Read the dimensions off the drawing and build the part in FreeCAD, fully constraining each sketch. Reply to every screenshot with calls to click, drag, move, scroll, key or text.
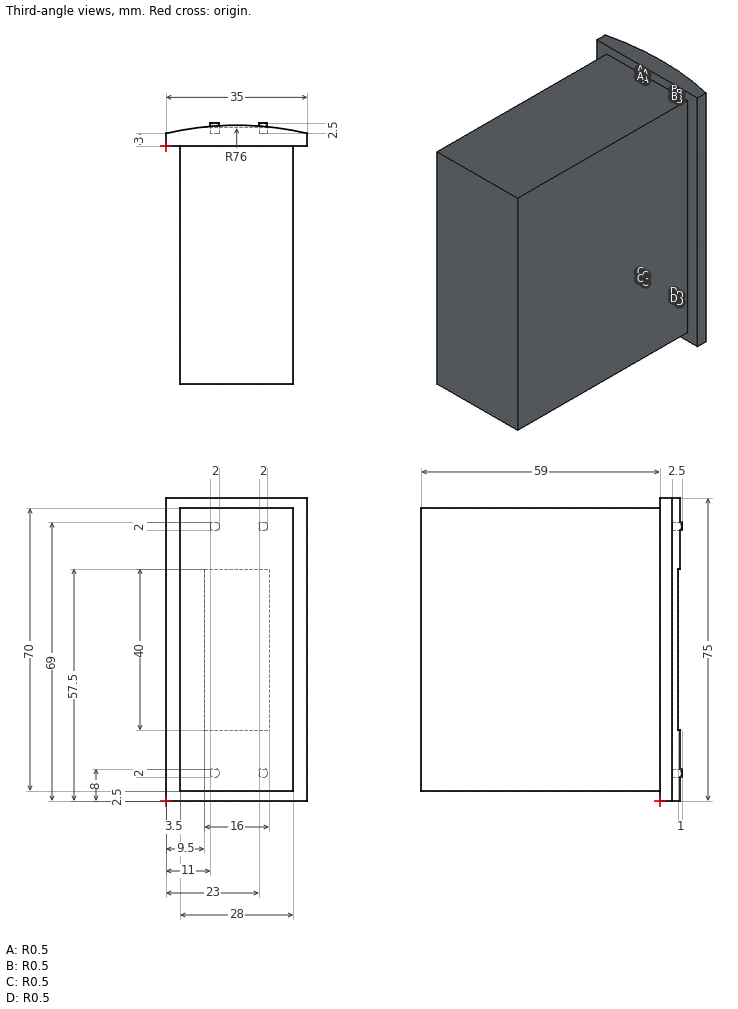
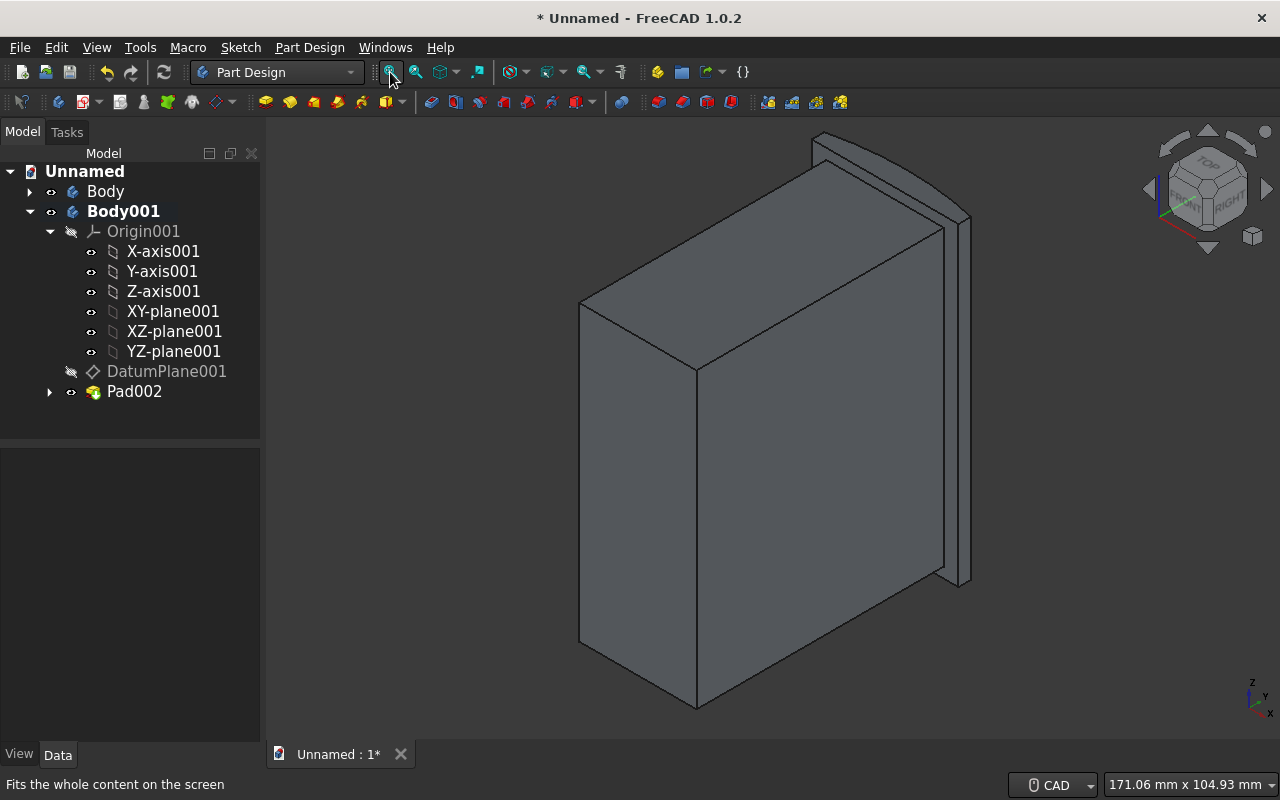
scroll(876, 184, up, 5)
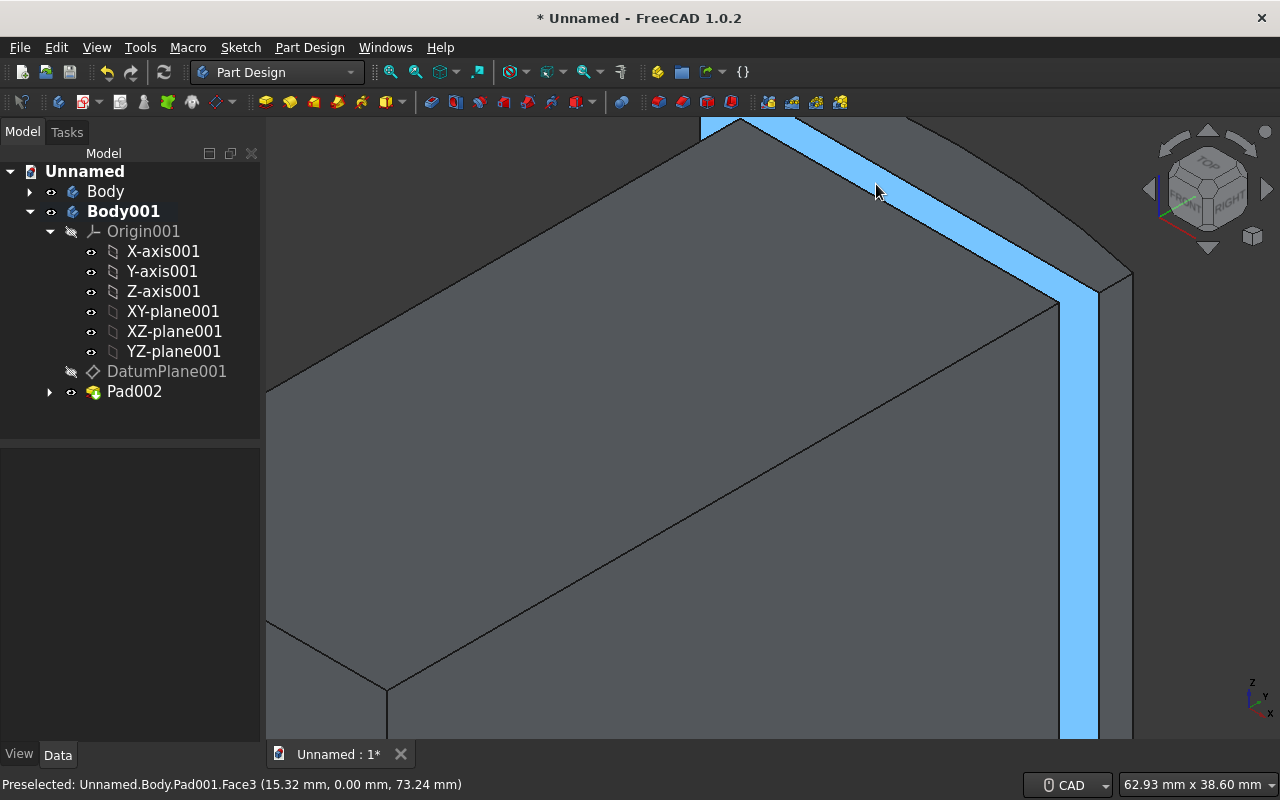
key(v)
key(f)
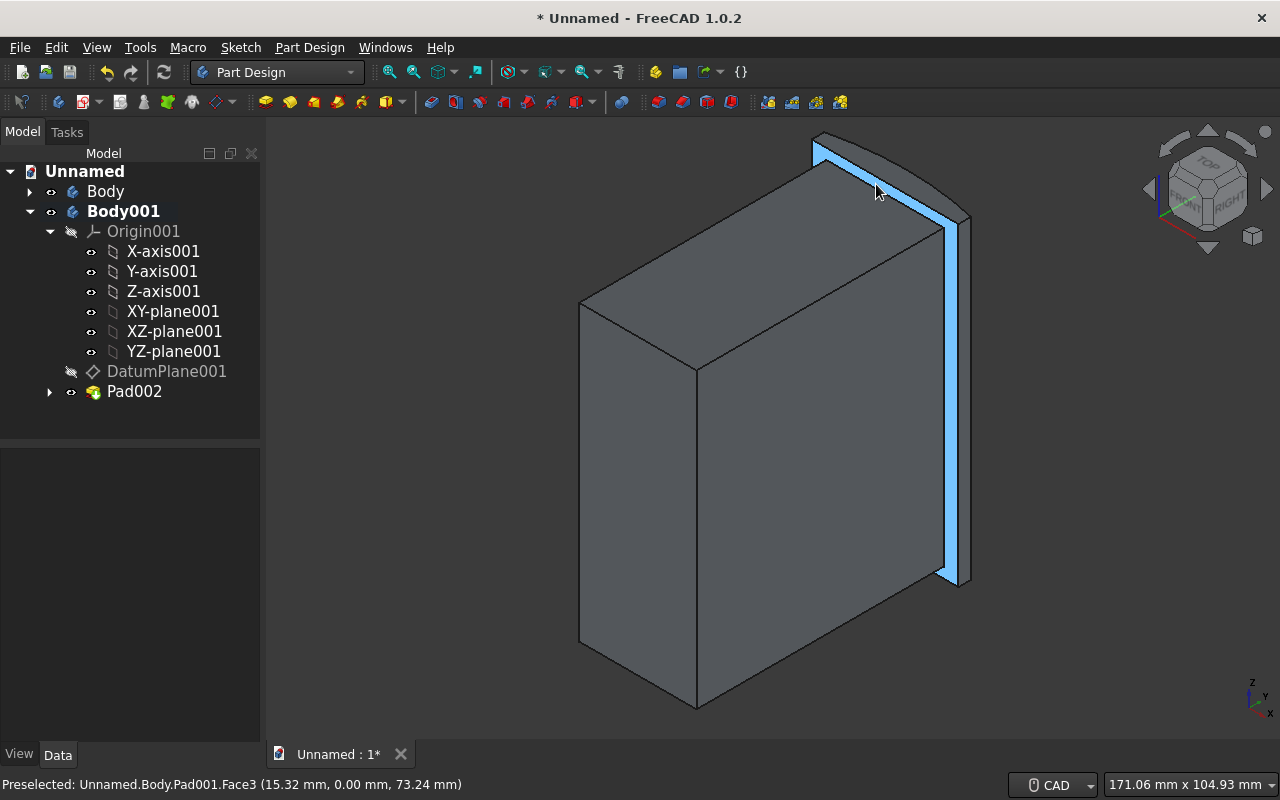
key(2)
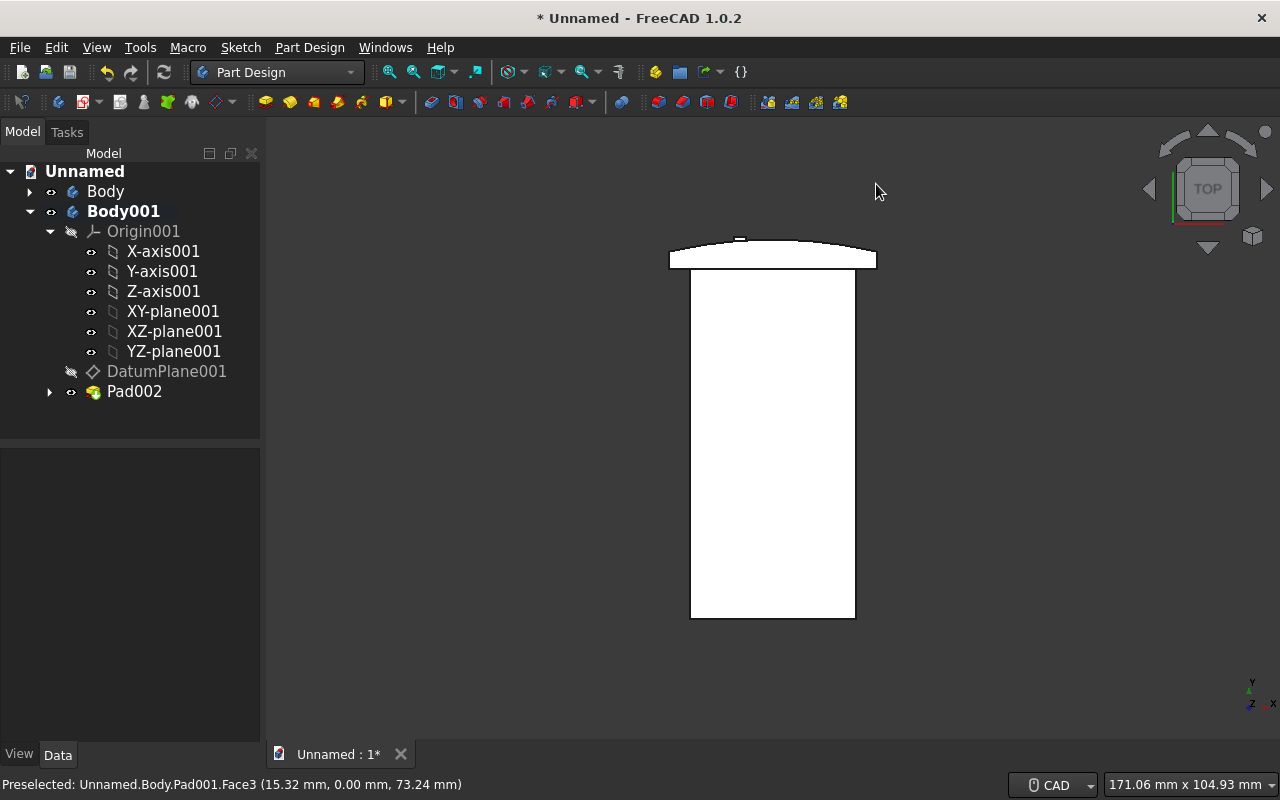
key(v)
key(f)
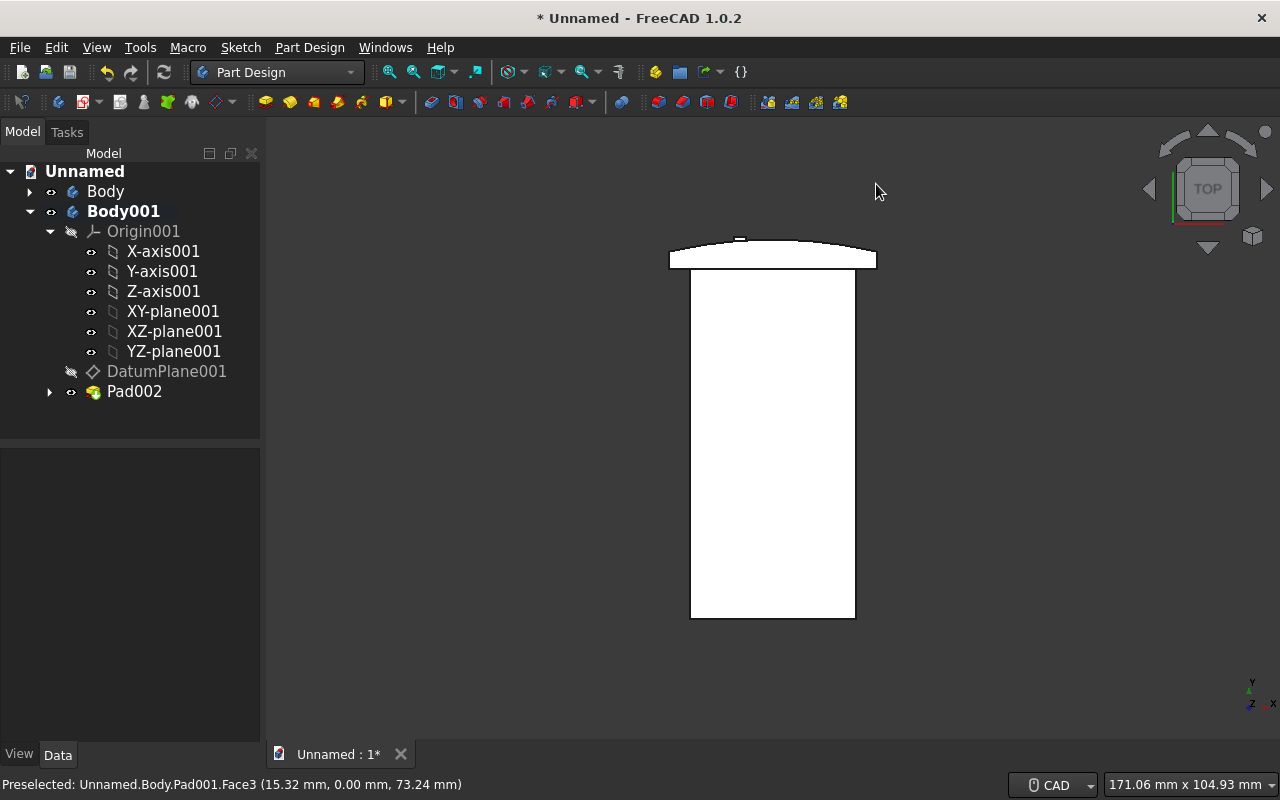
scroll(734, 243, up, 5)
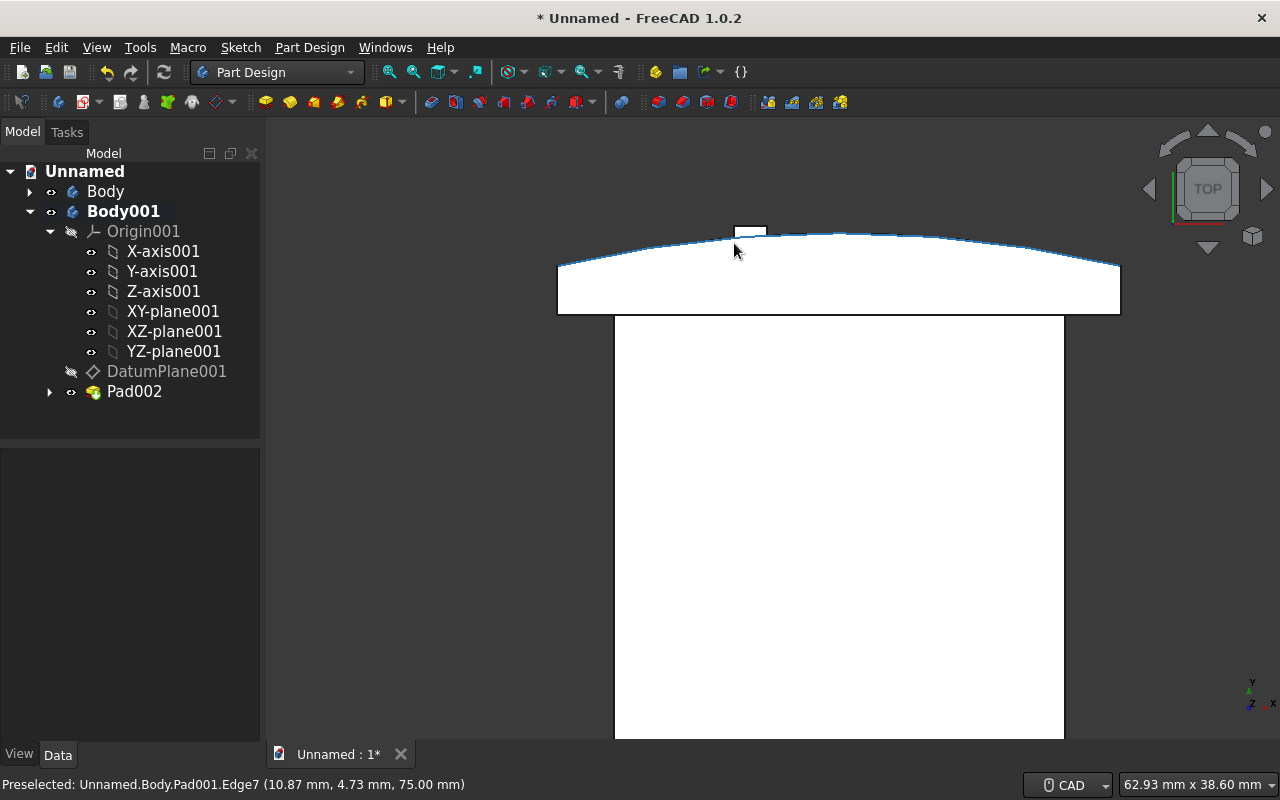
key(v)
key(f)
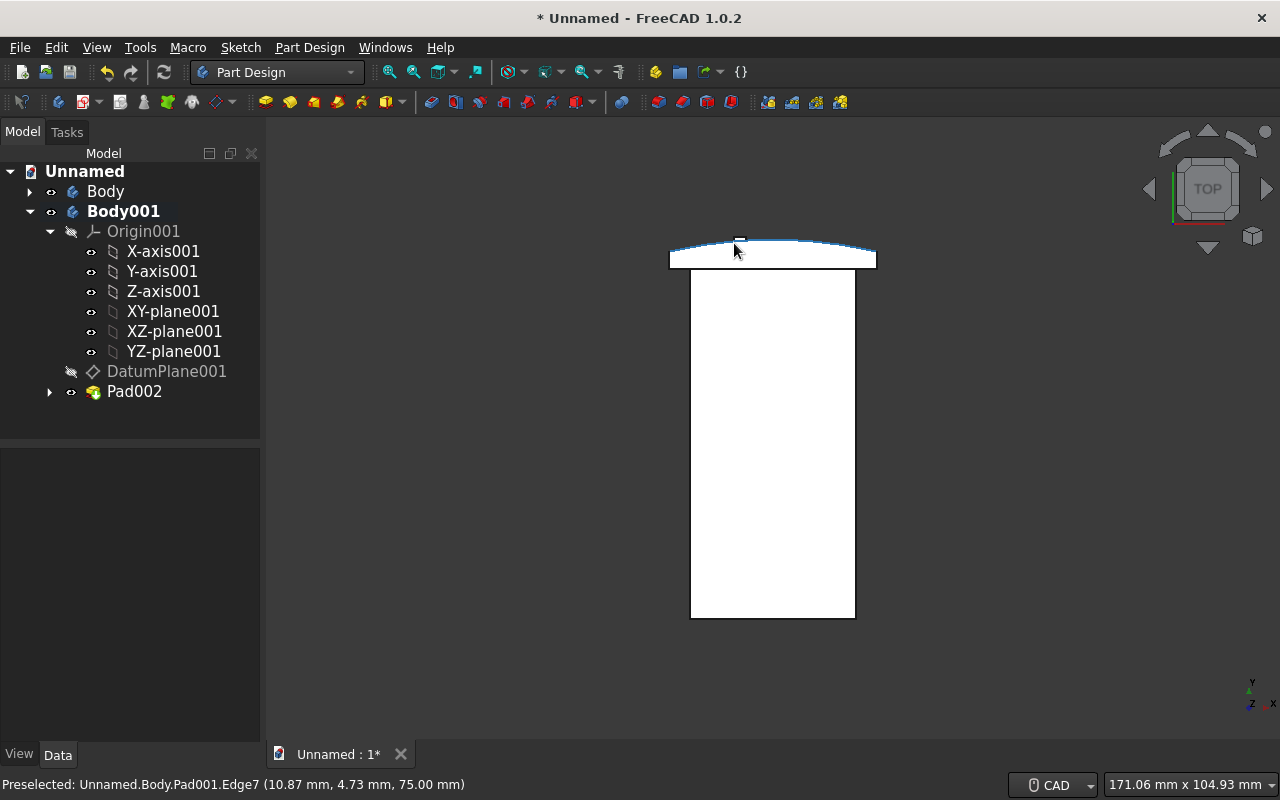
key(1)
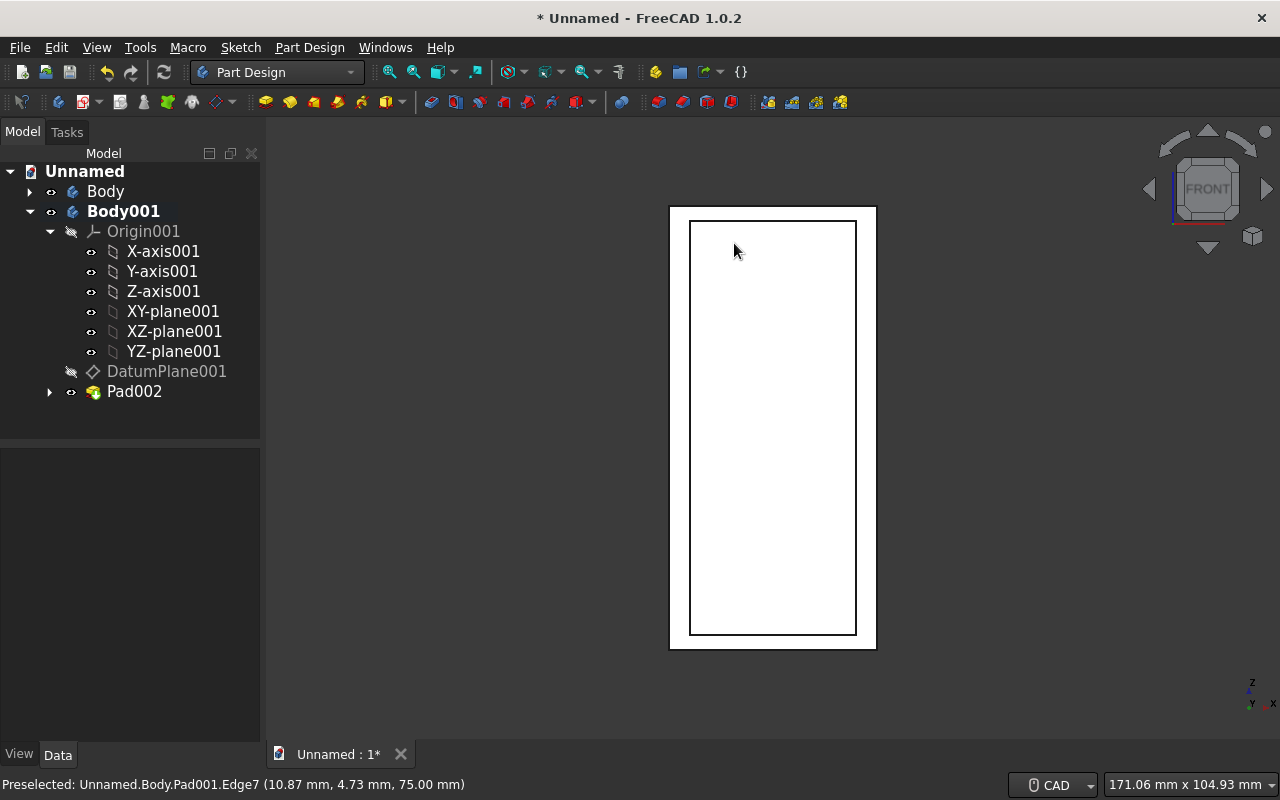
click(390, 72)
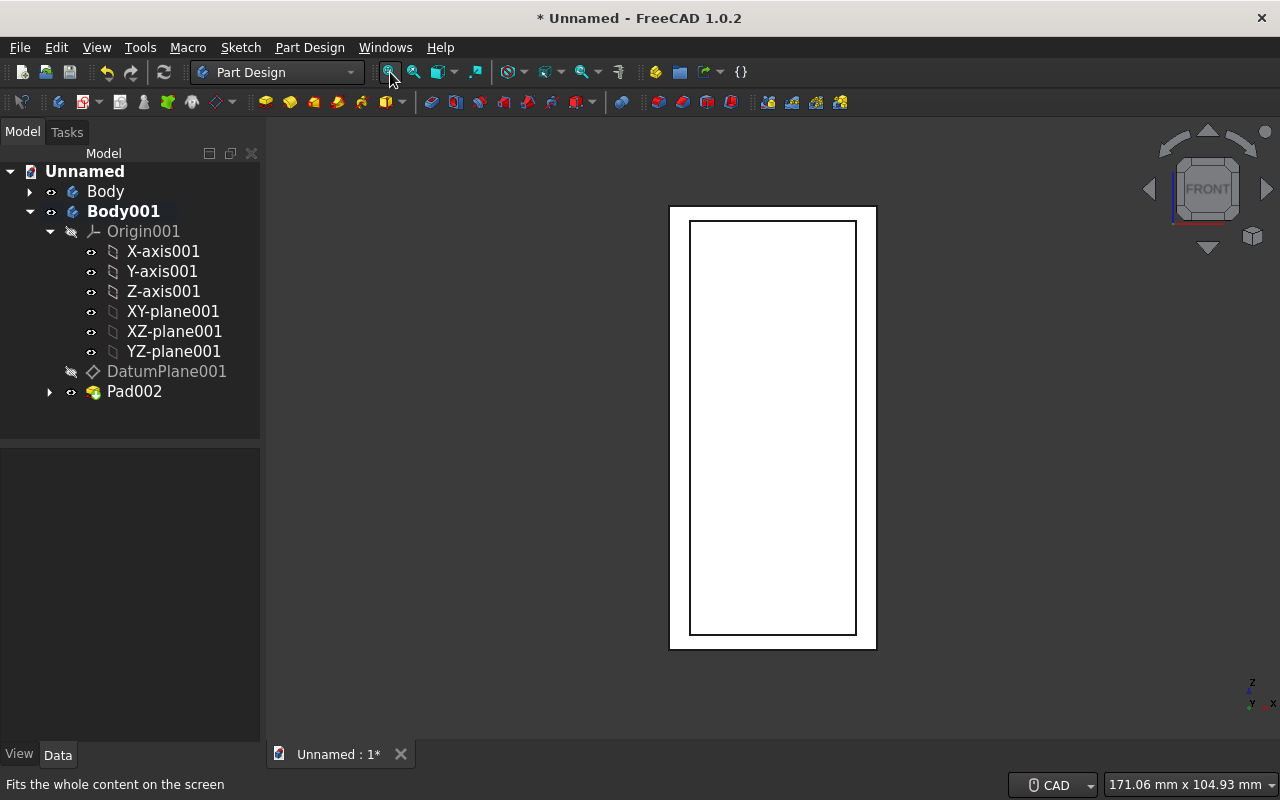
scroll(734, 240, up, 5)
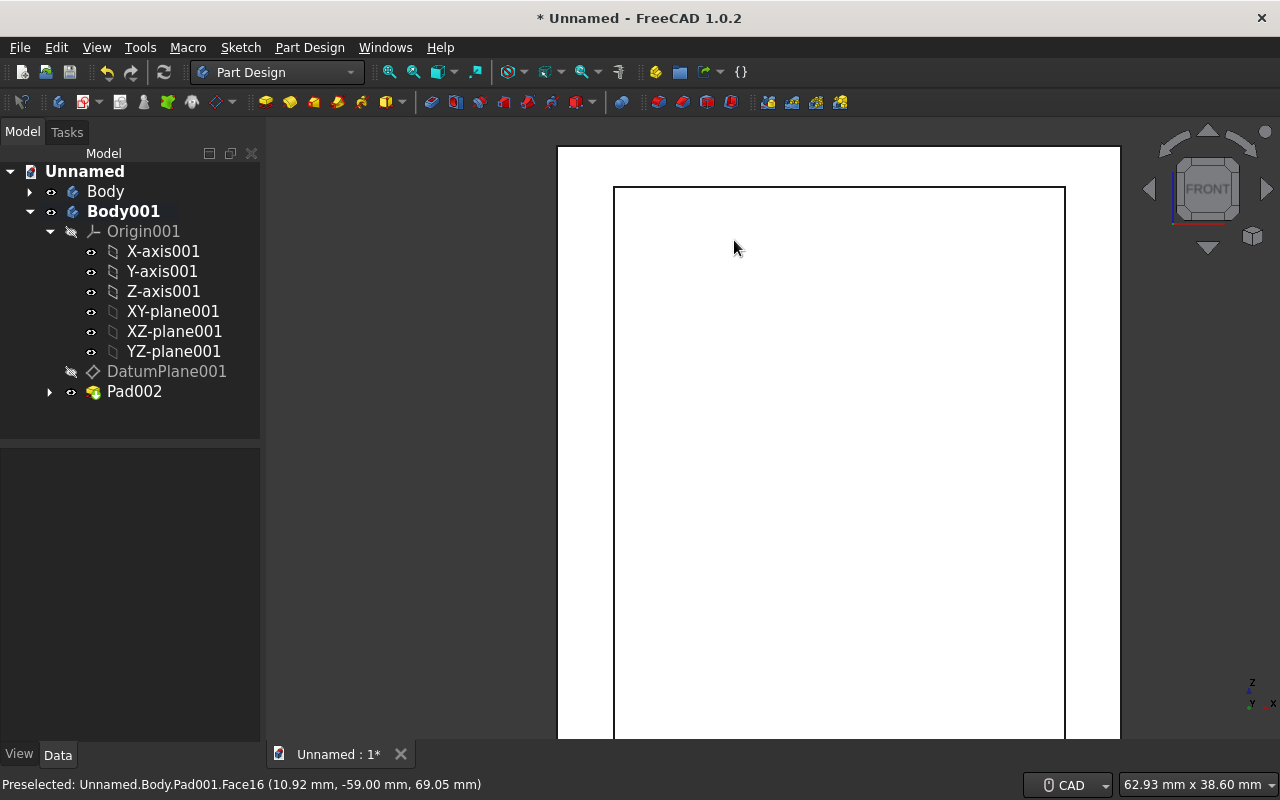
click(390, 72)